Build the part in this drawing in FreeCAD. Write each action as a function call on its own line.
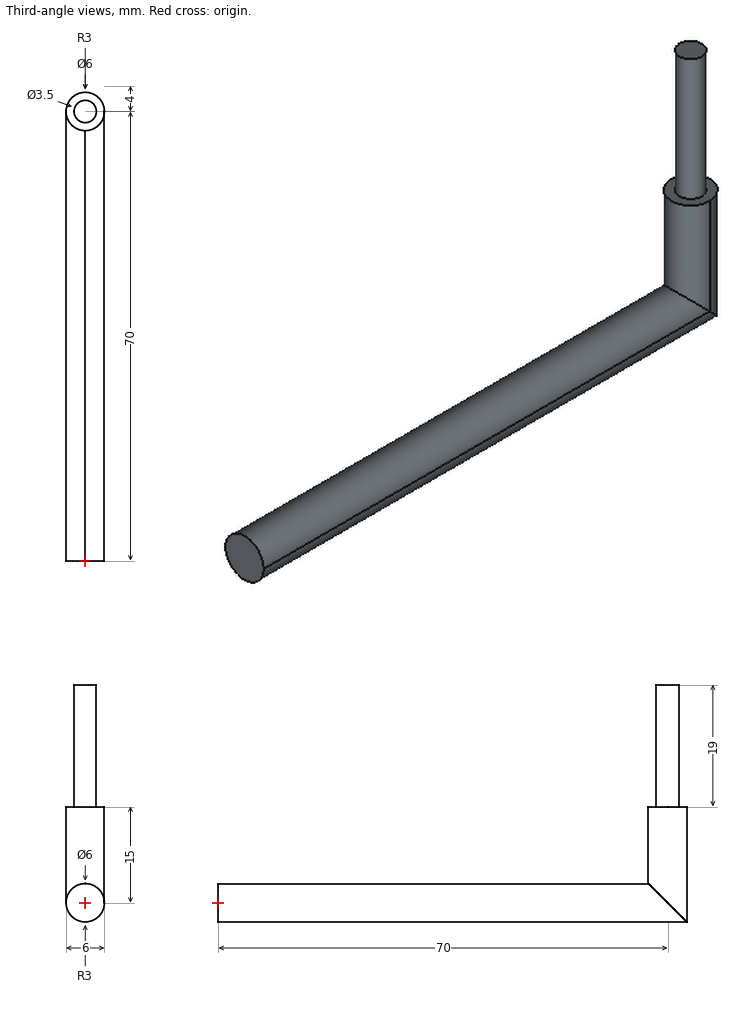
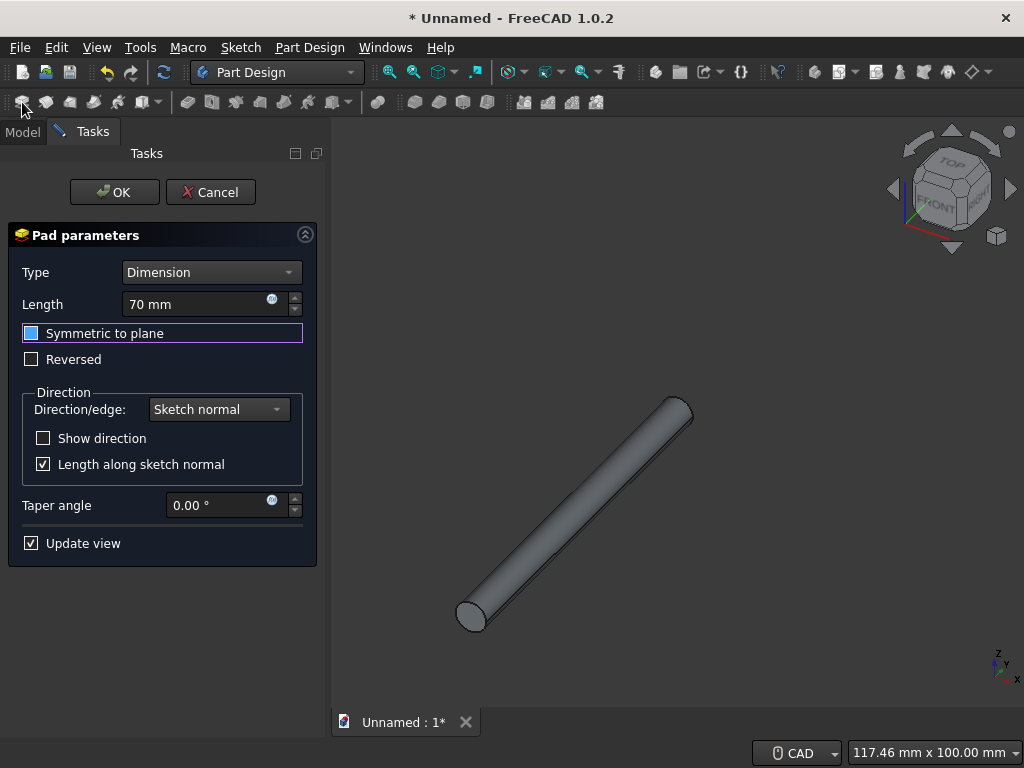
click(30, 359)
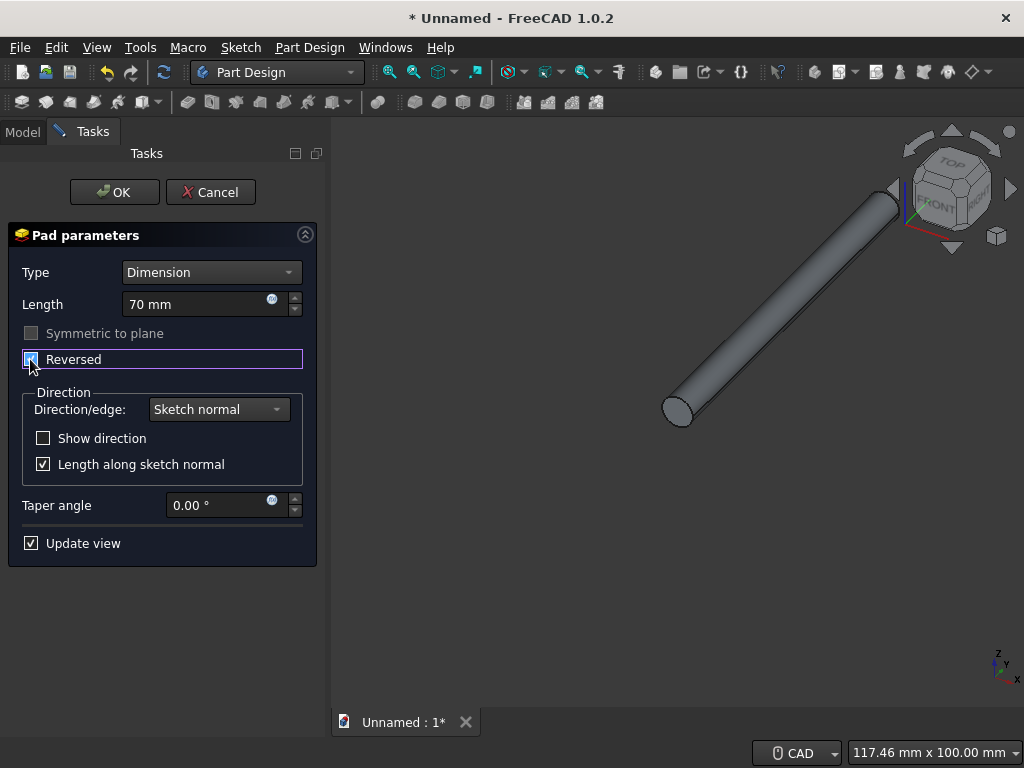
click(115, 192)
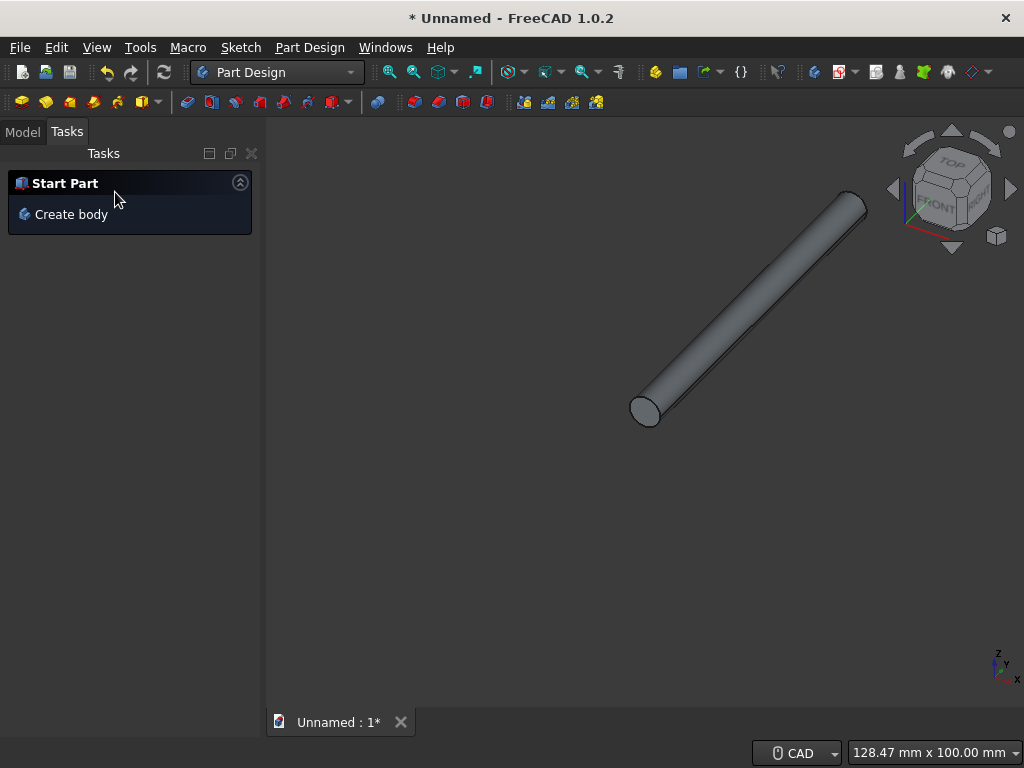
key(v)
key(f)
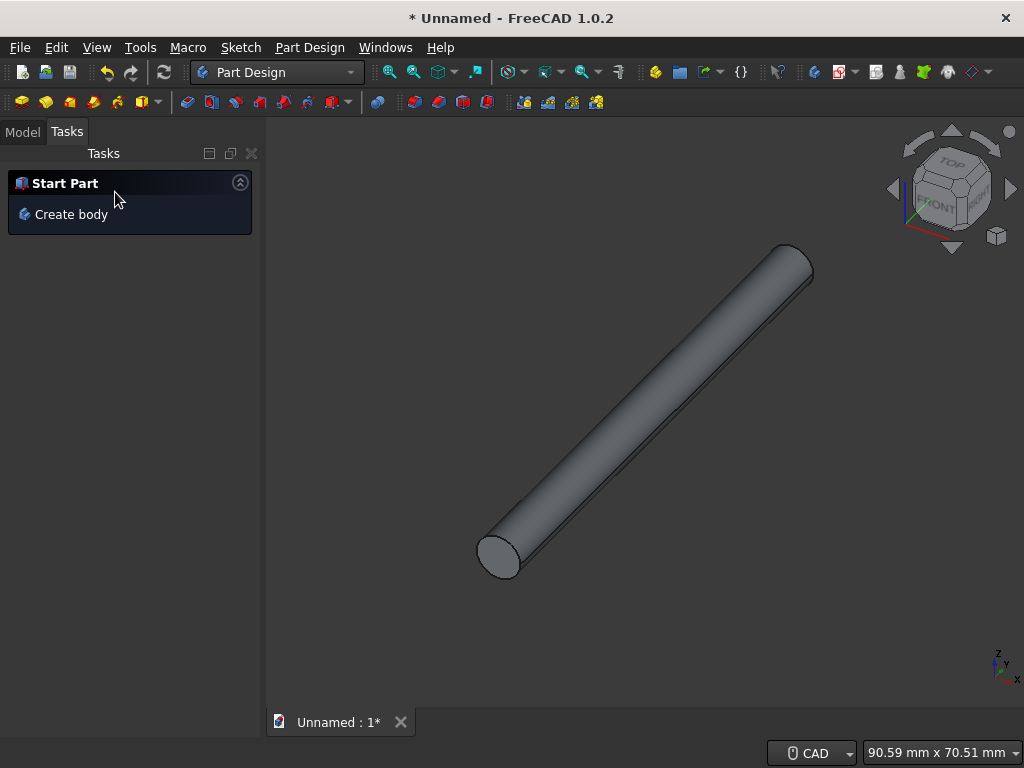
click(840, 72)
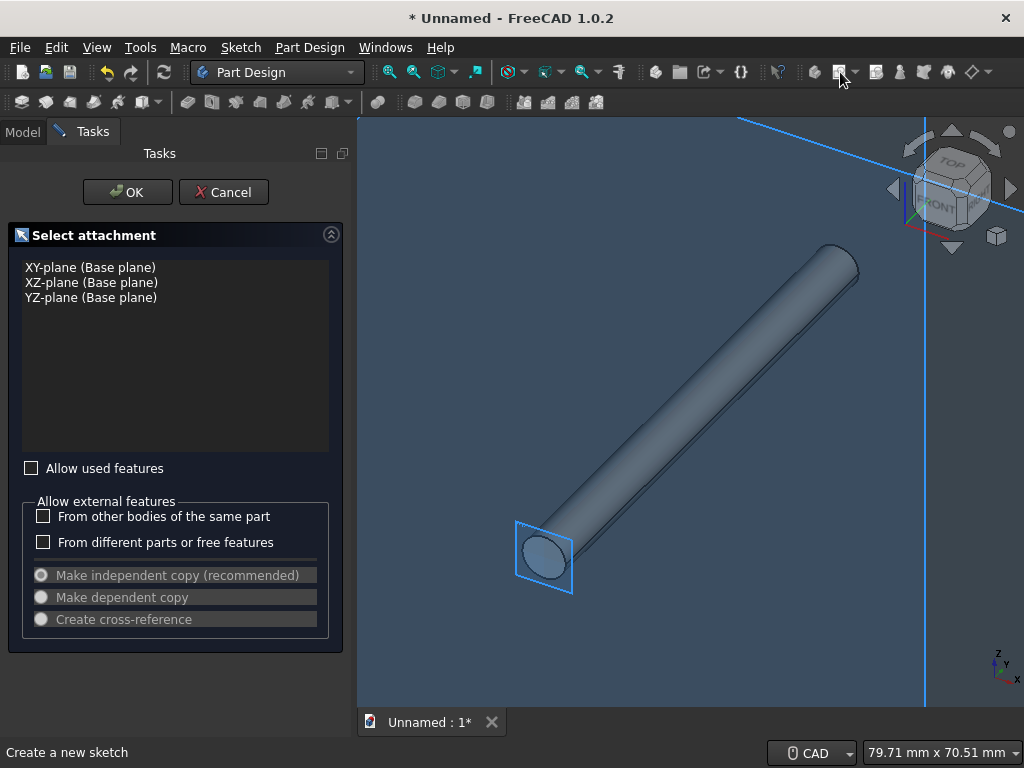
click(82, 268)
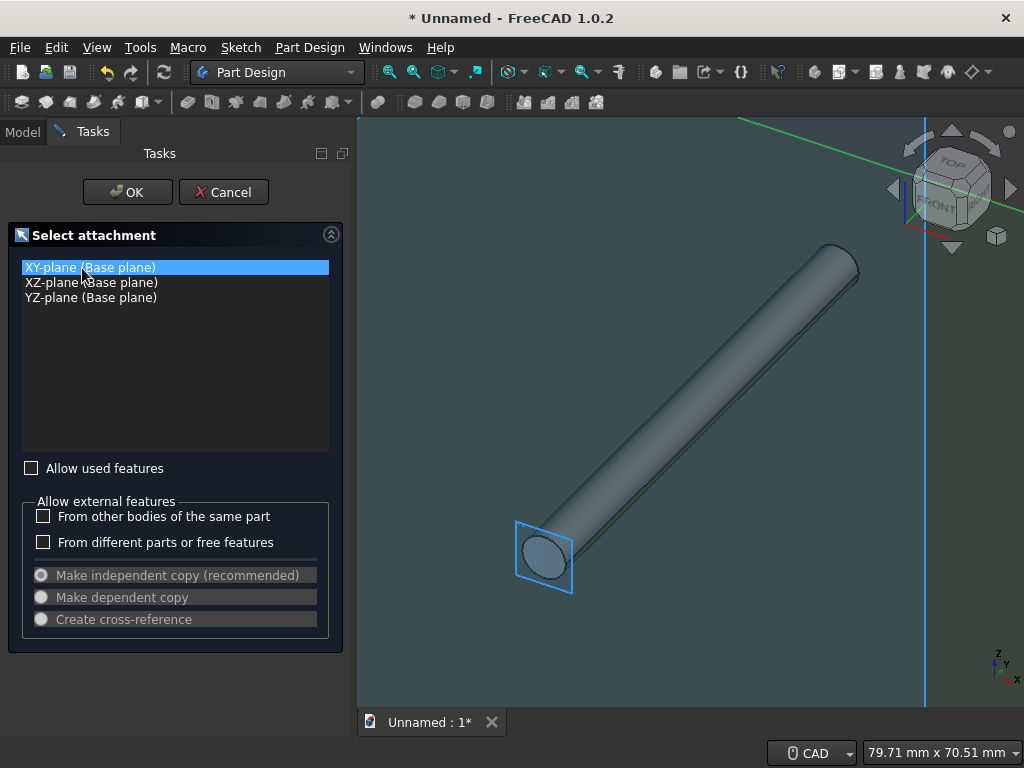
click(128, 192)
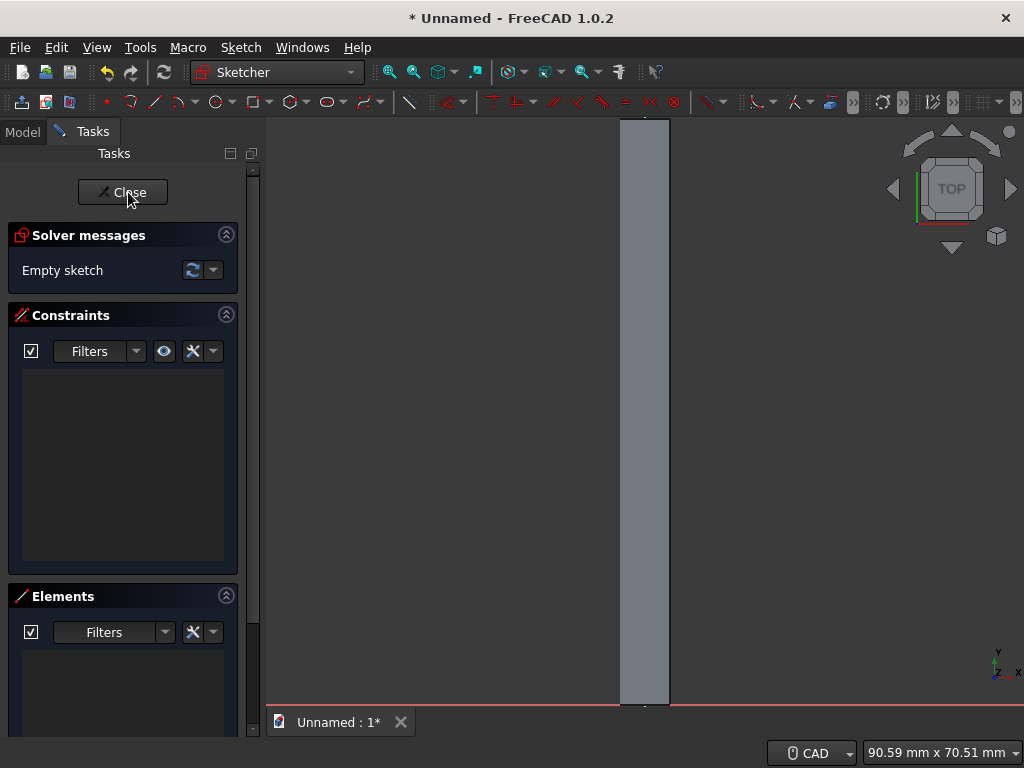
key(q)
key(s)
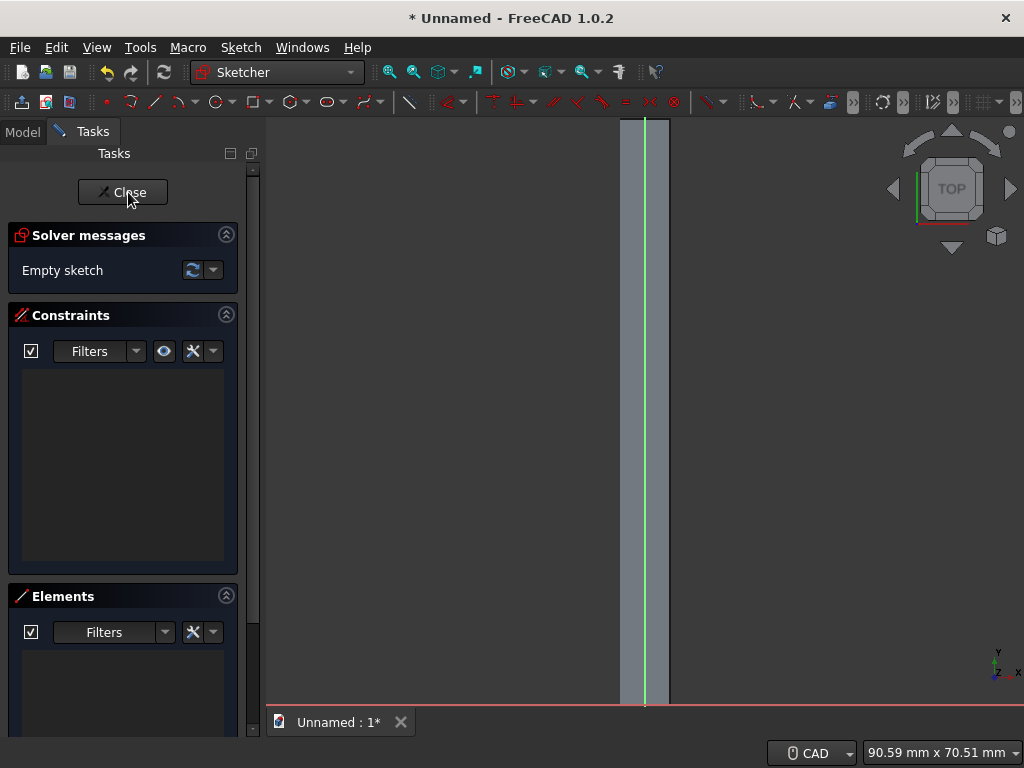
scroll(576, 412, down, 5)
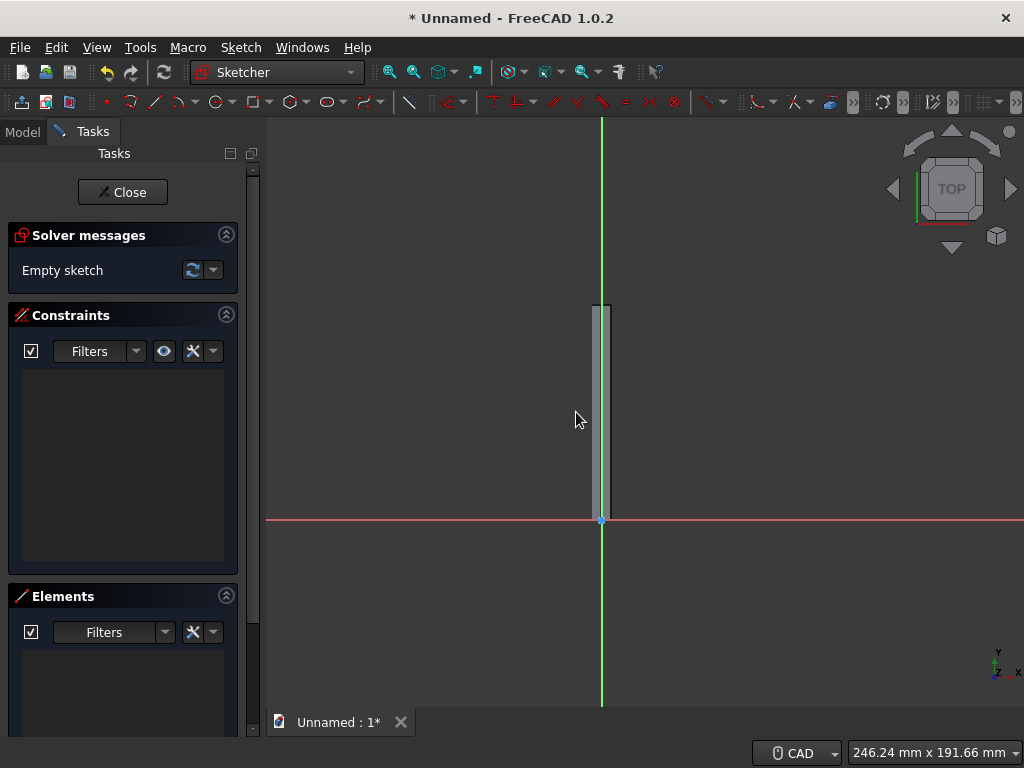
scroll(603, 299, up, 15)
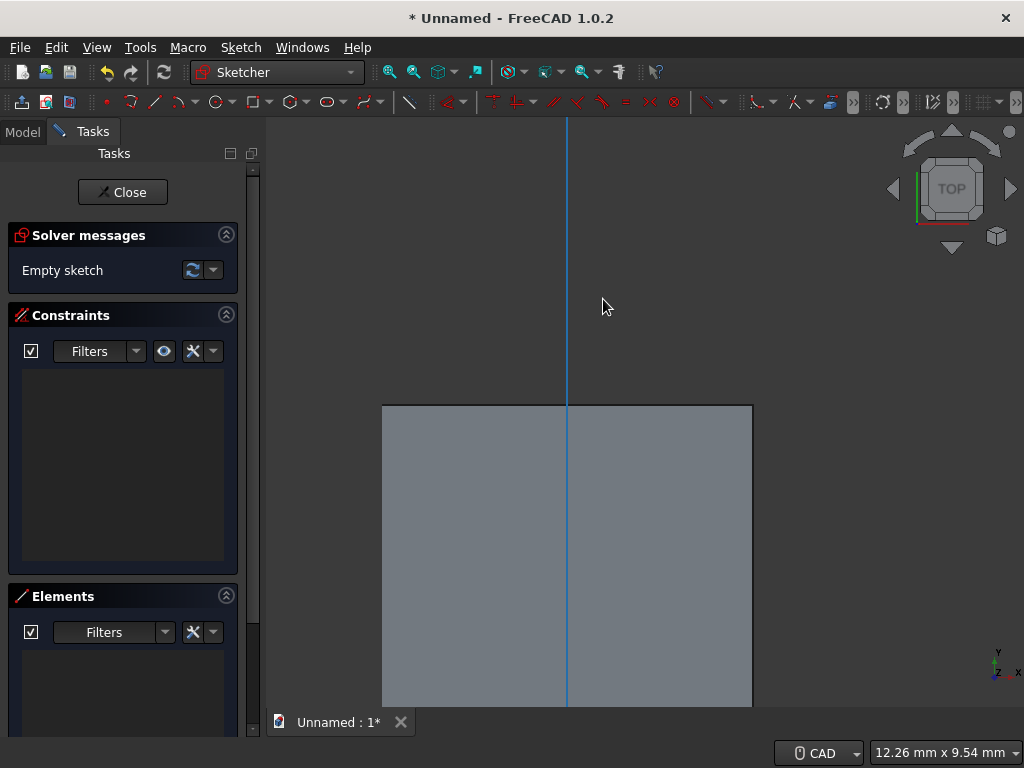
key(g)
key(c)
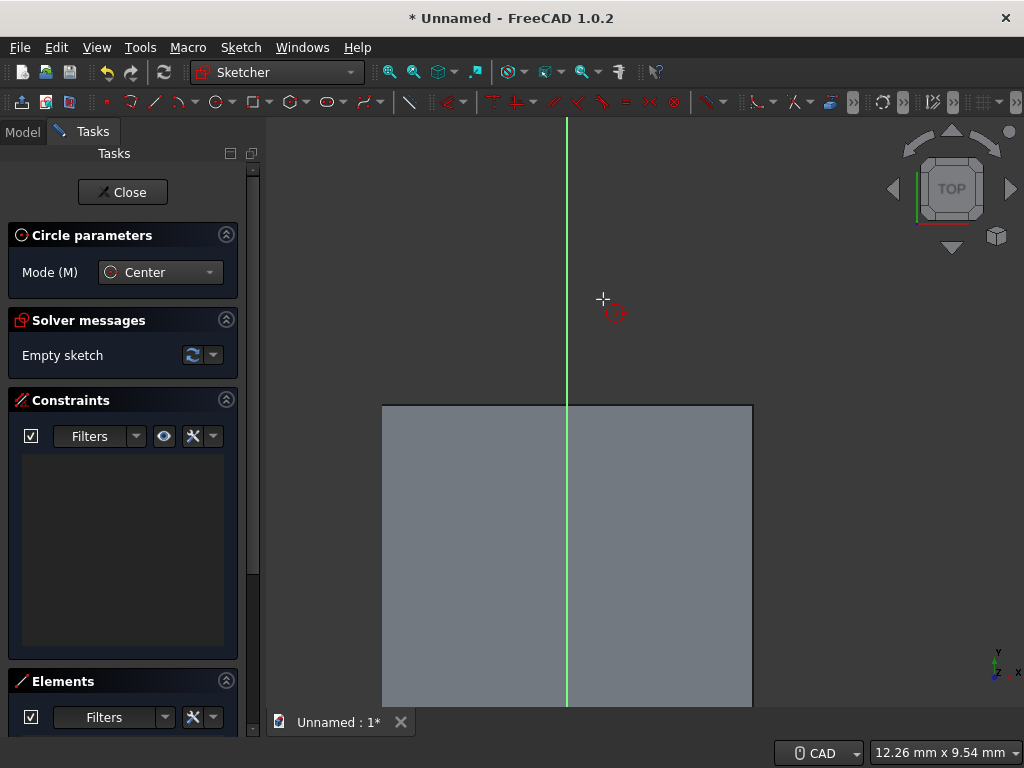
click(567, 405)
click(698, 274)
key(Escape)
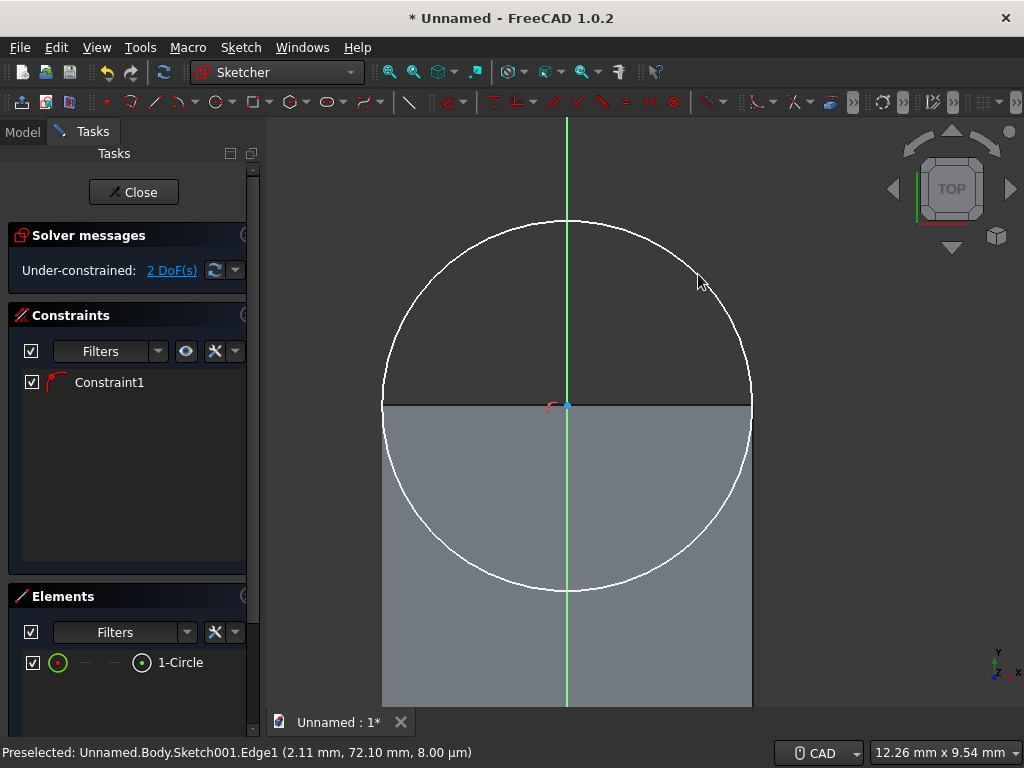
key(d)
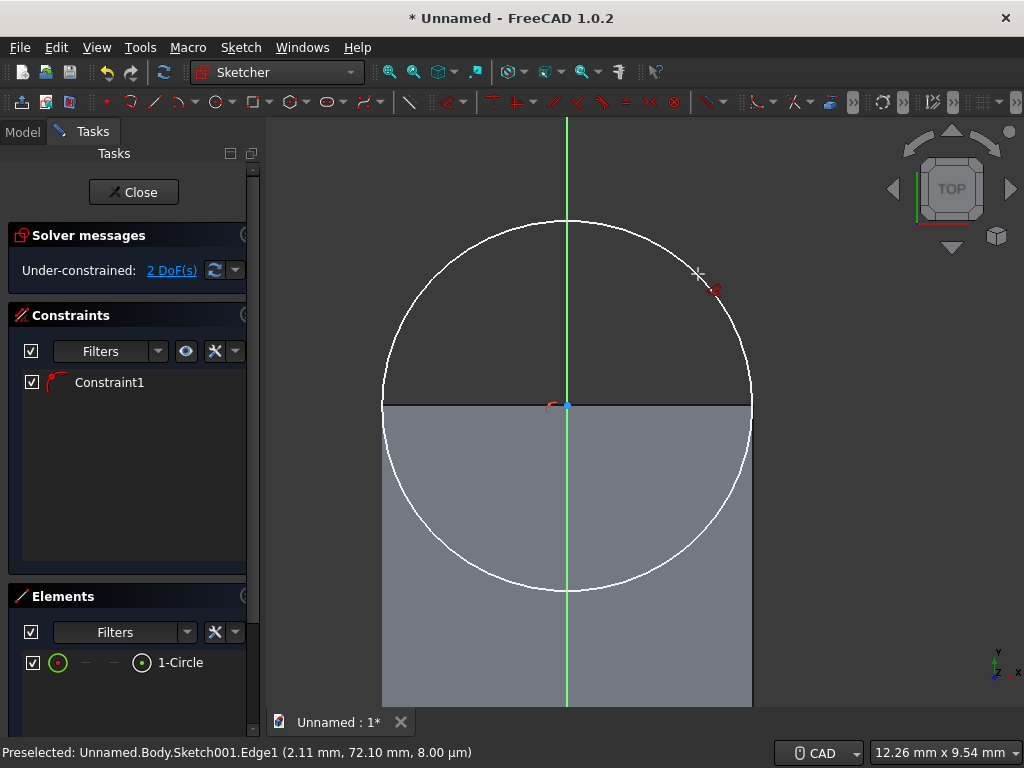
click(698, 275)
click(721, 252)